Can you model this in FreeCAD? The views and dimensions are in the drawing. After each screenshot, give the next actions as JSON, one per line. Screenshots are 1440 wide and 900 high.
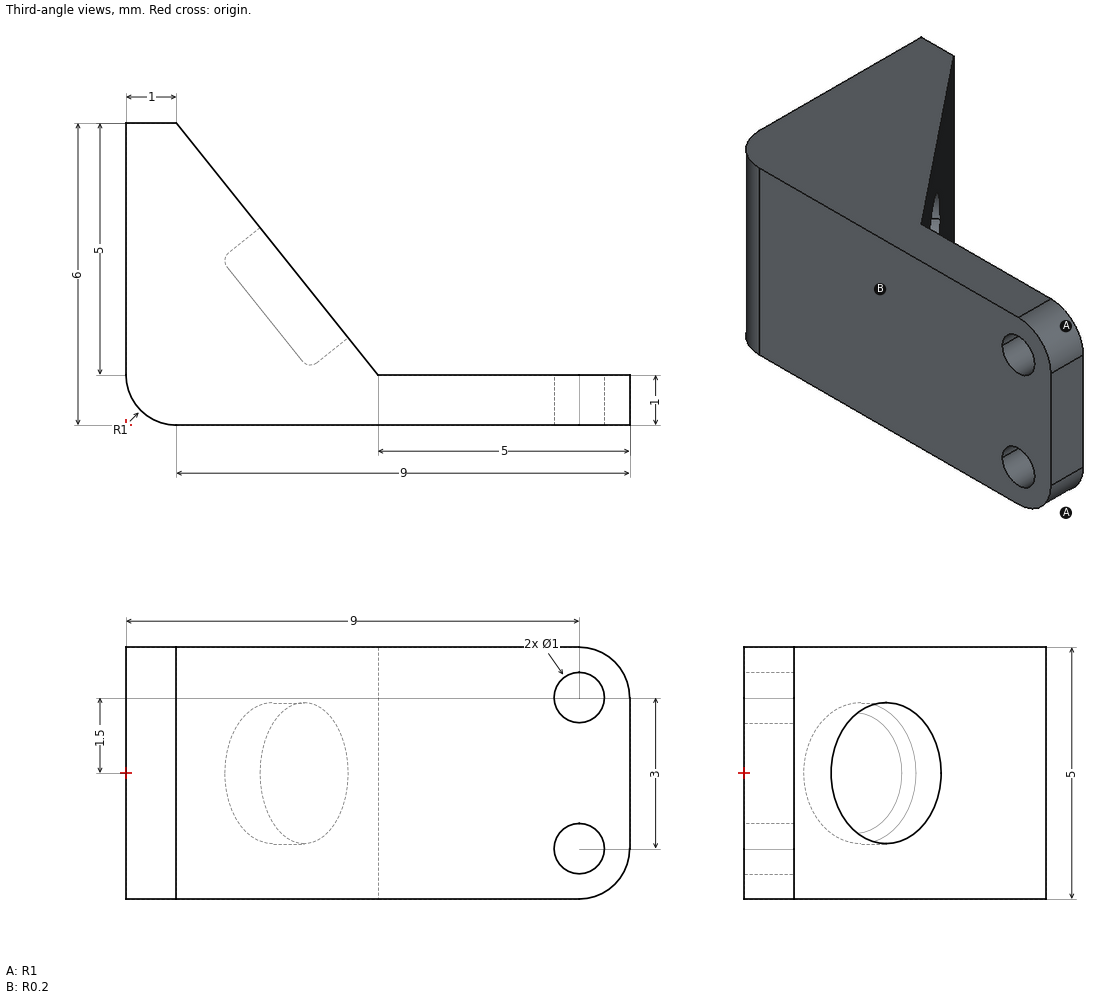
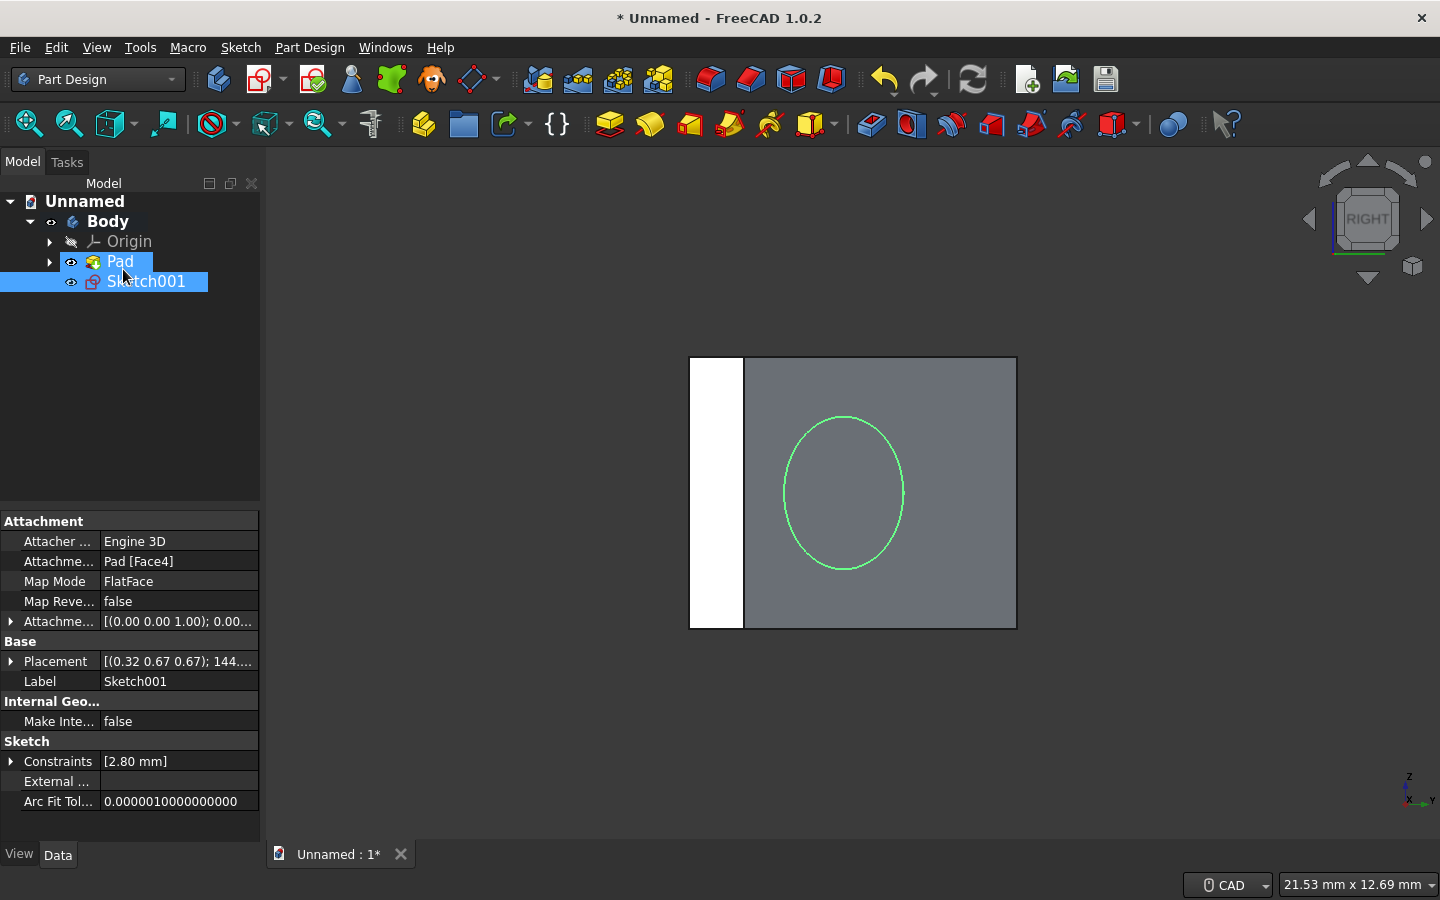
{"action": "left_click", "coordinate": [872, 124]}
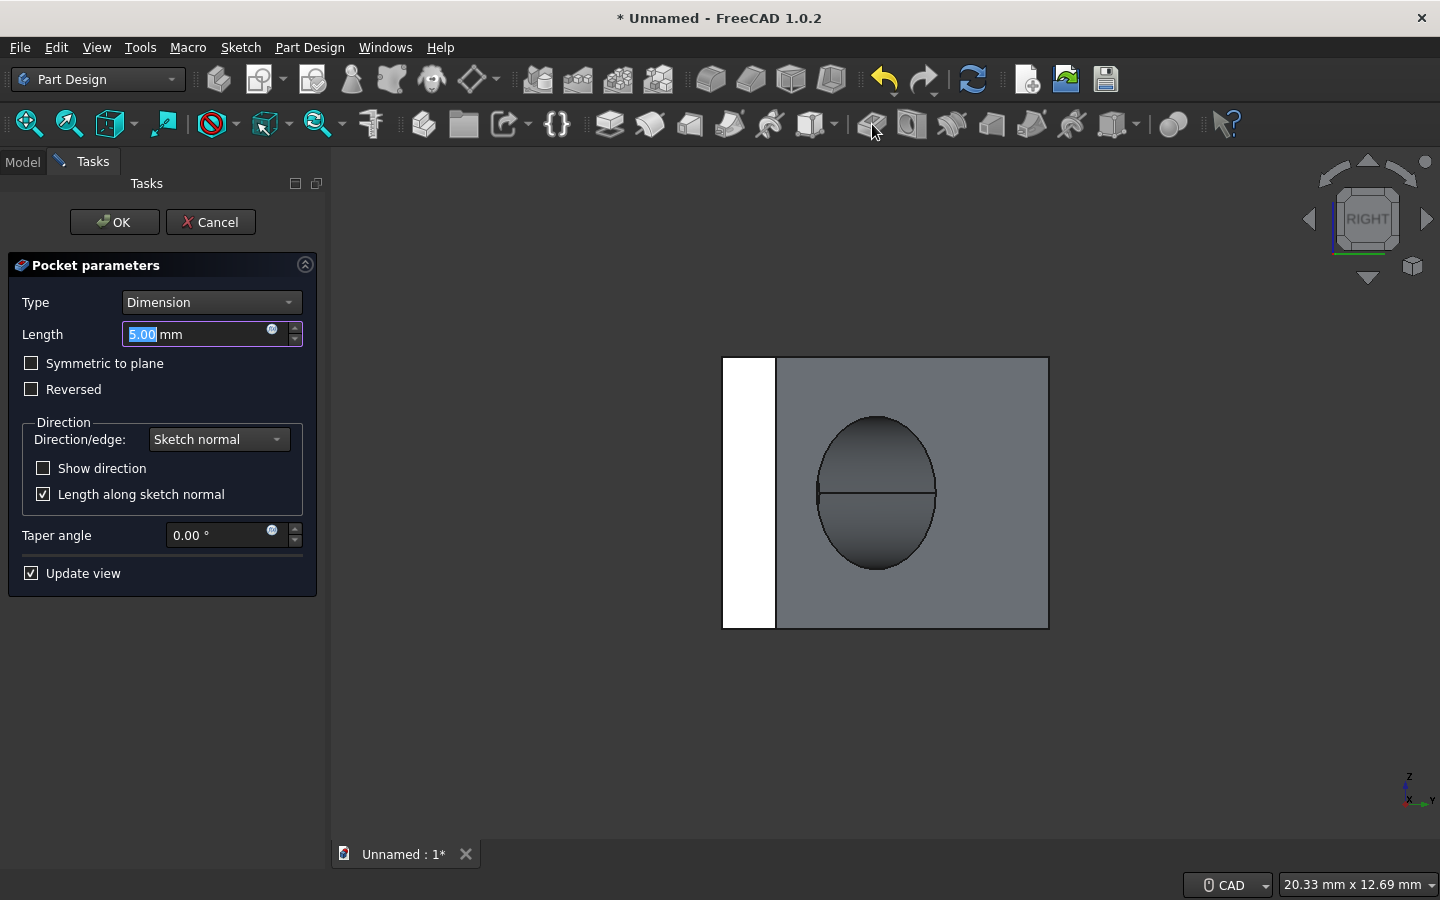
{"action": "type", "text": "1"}
{"action": "key", "text": "Tab"}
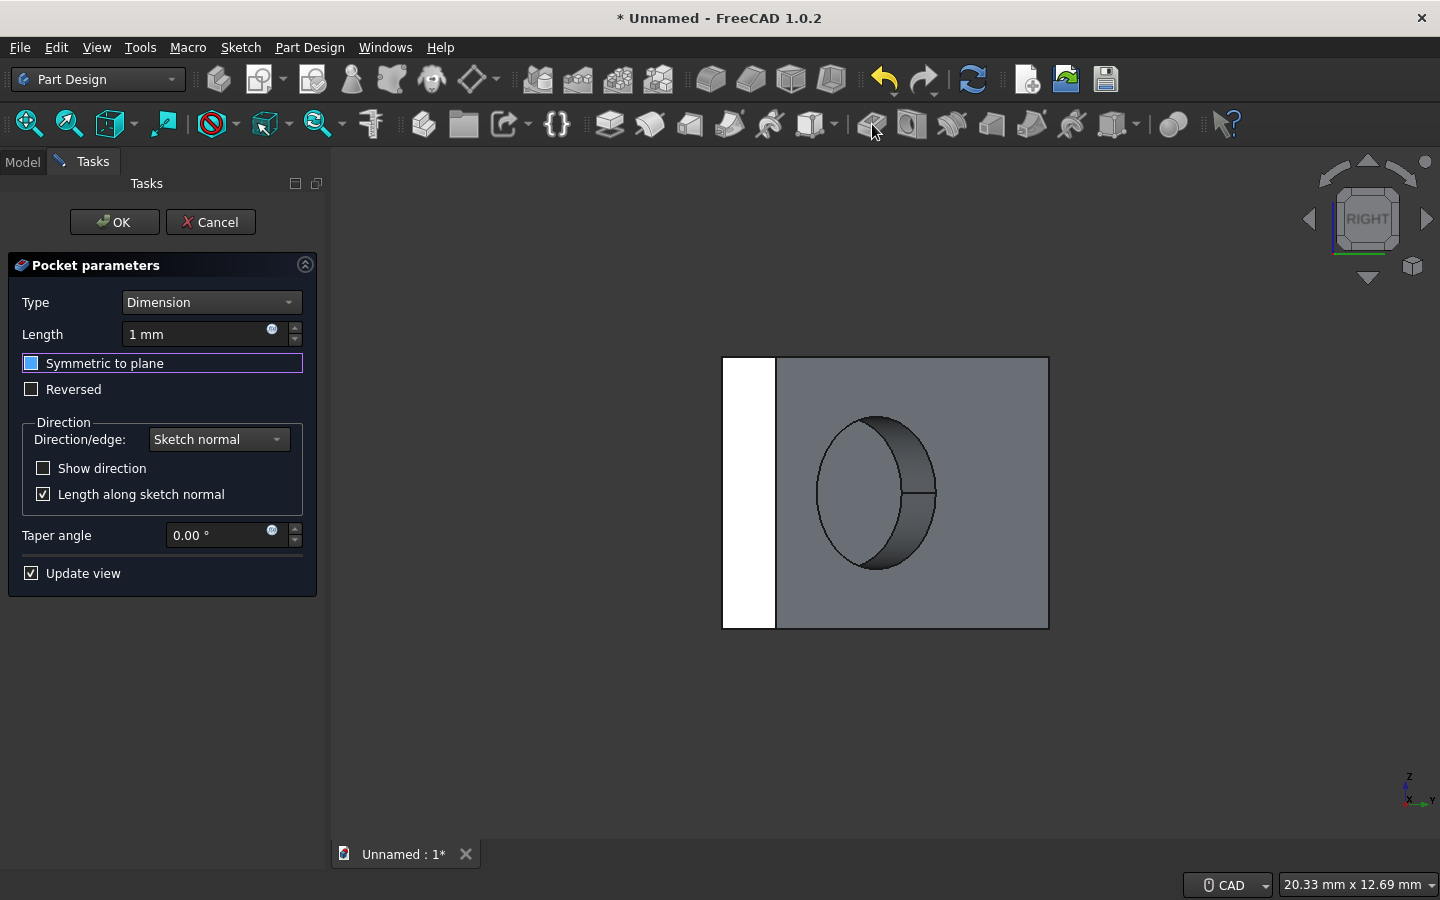
{"action": "left_click", "coordinate": [115, 222]}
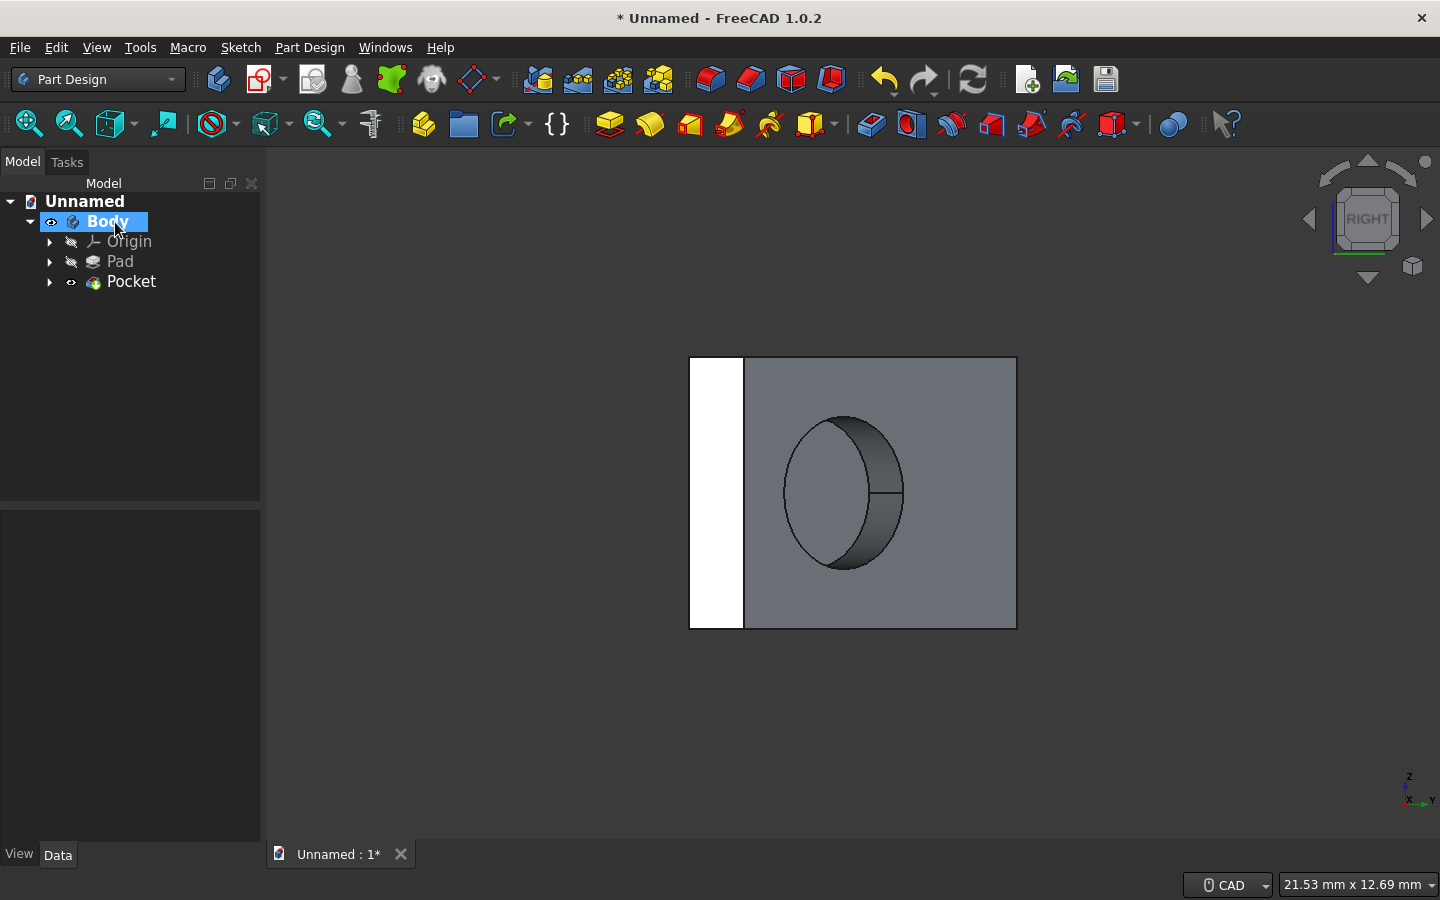
{"action": "left_click", "coordinate": [30, 124]}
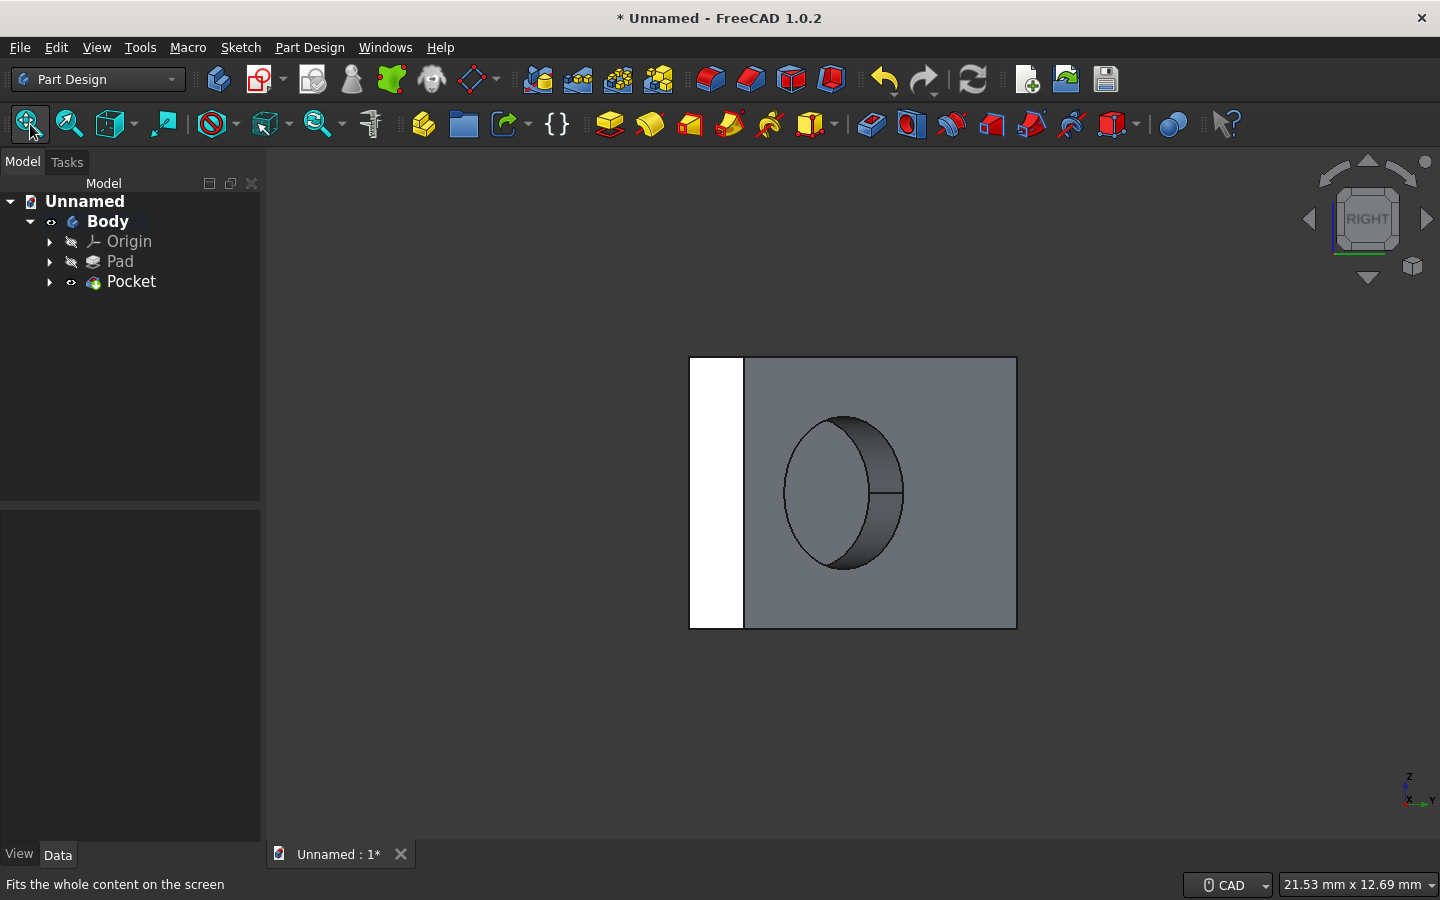
{"action": "key", "text": "4"}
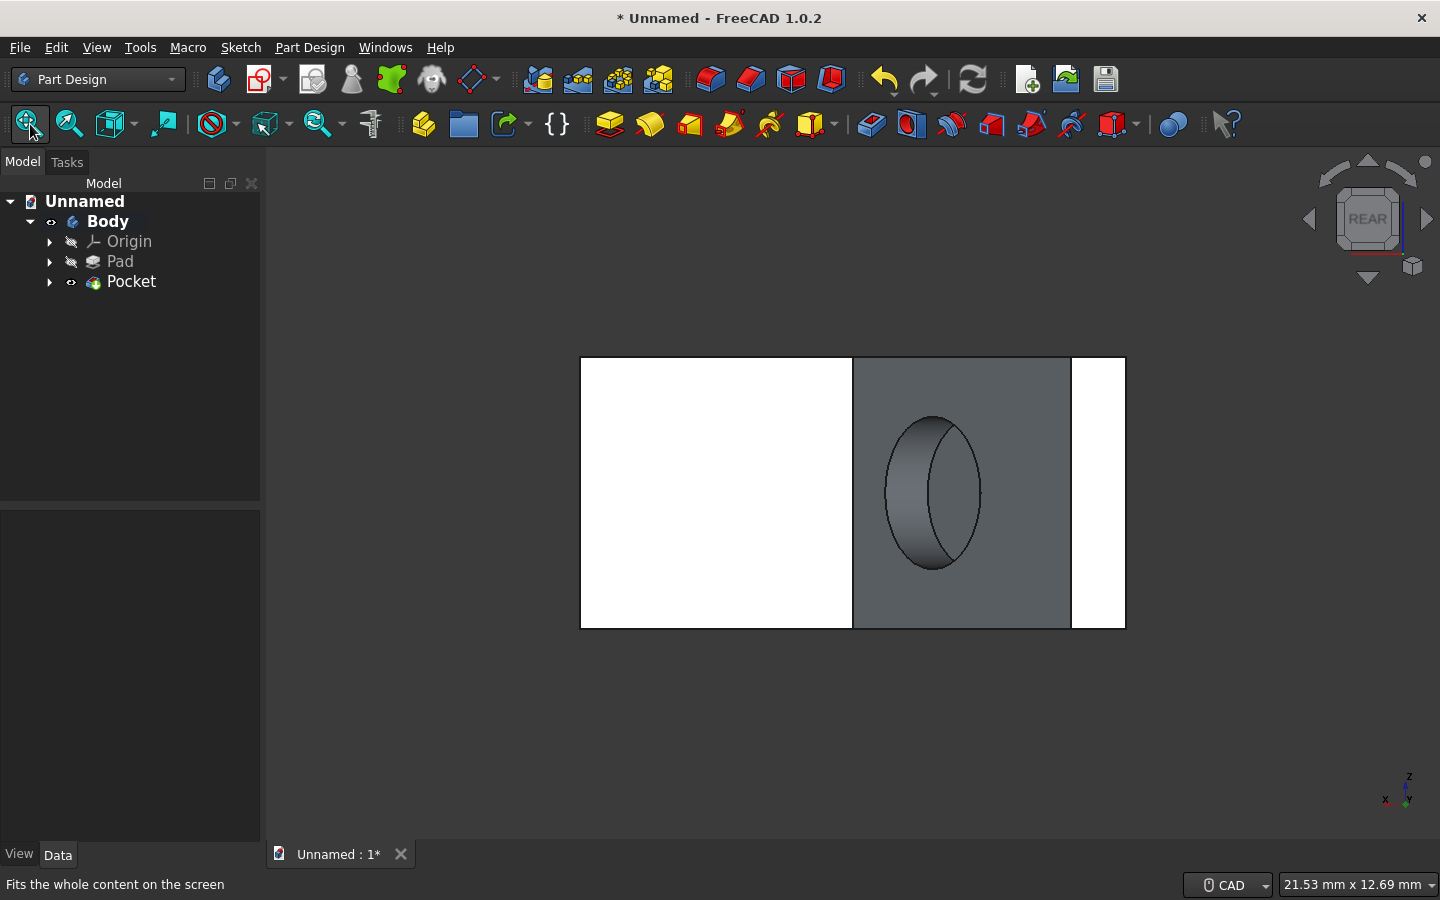
{"action": "left_click", "coordinate": [717, 492]}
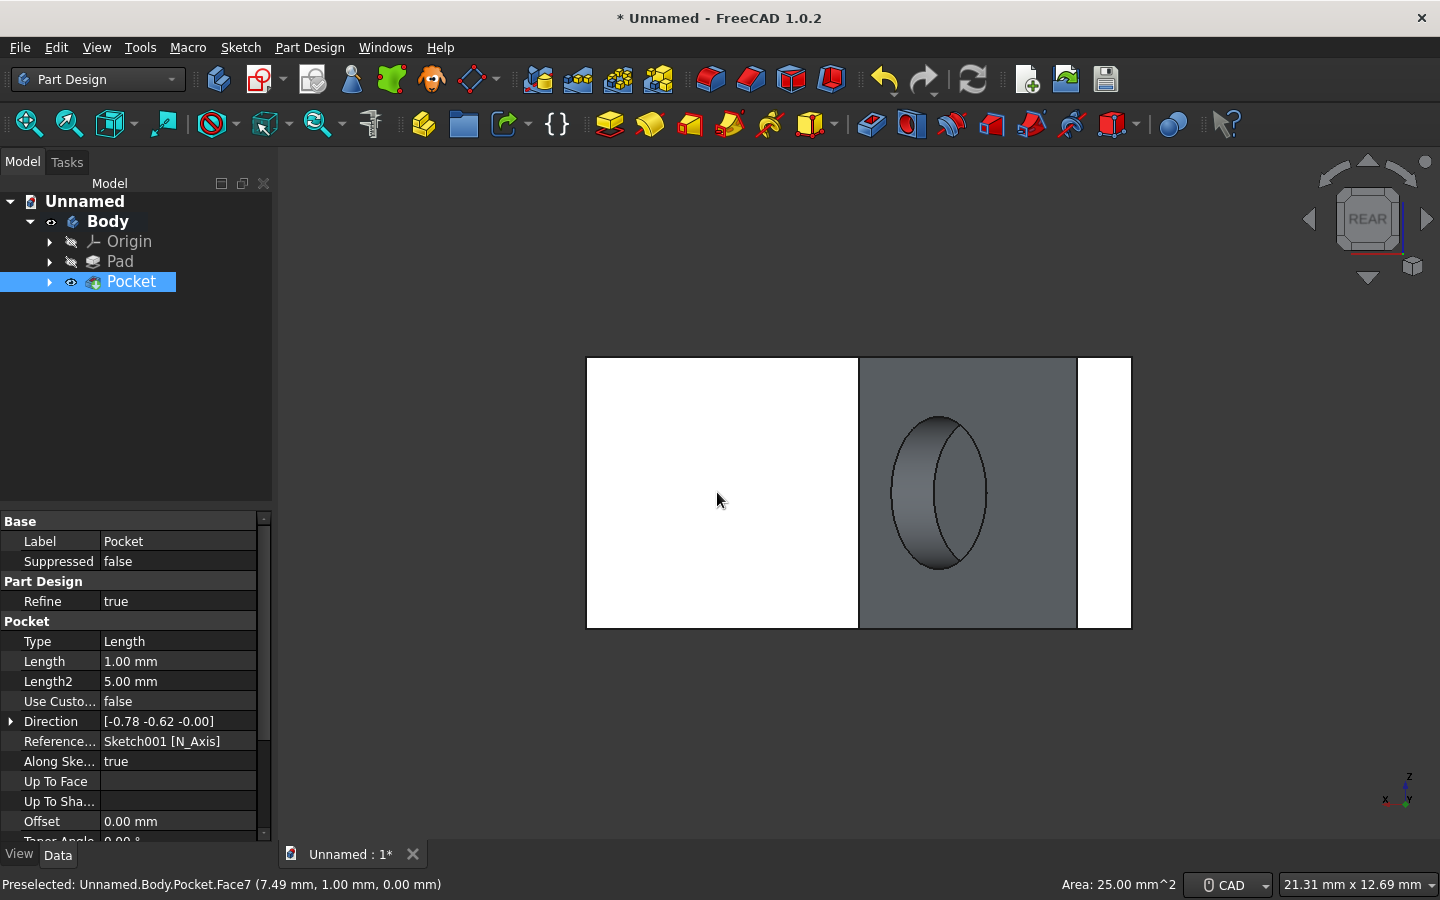
{"action": "left_click", "coordinate": [260, 80]}